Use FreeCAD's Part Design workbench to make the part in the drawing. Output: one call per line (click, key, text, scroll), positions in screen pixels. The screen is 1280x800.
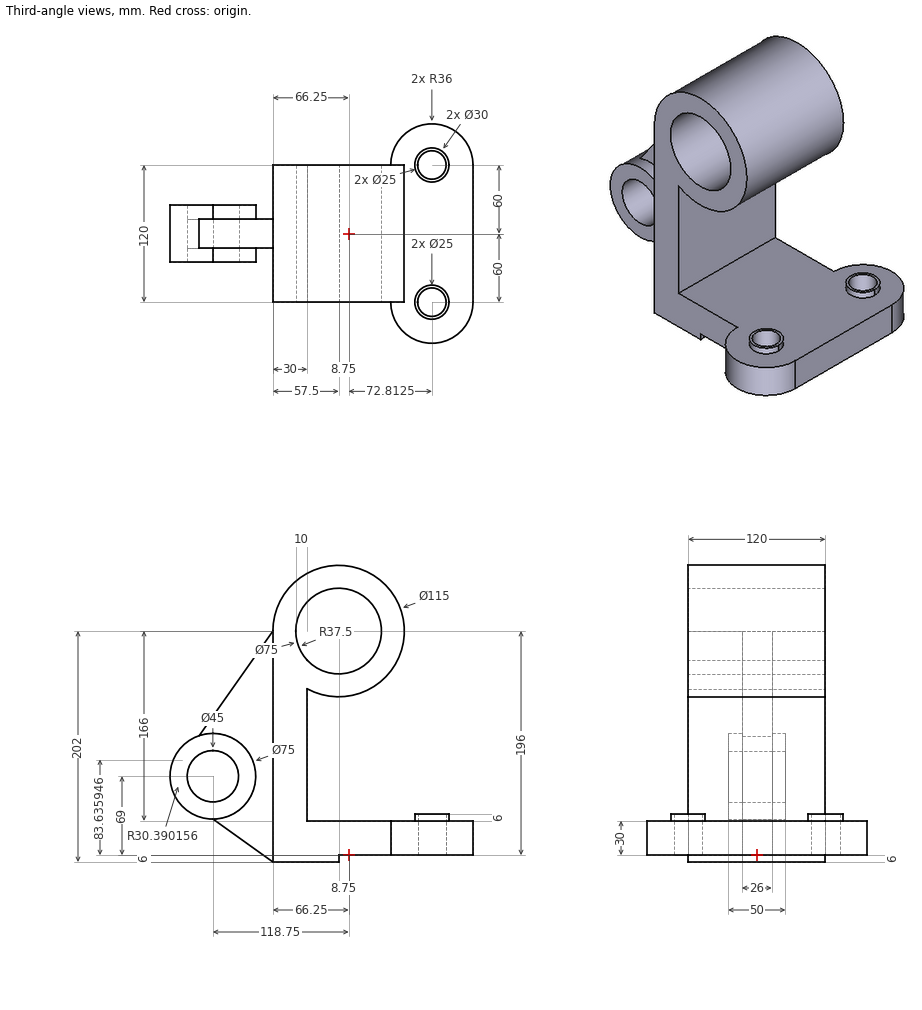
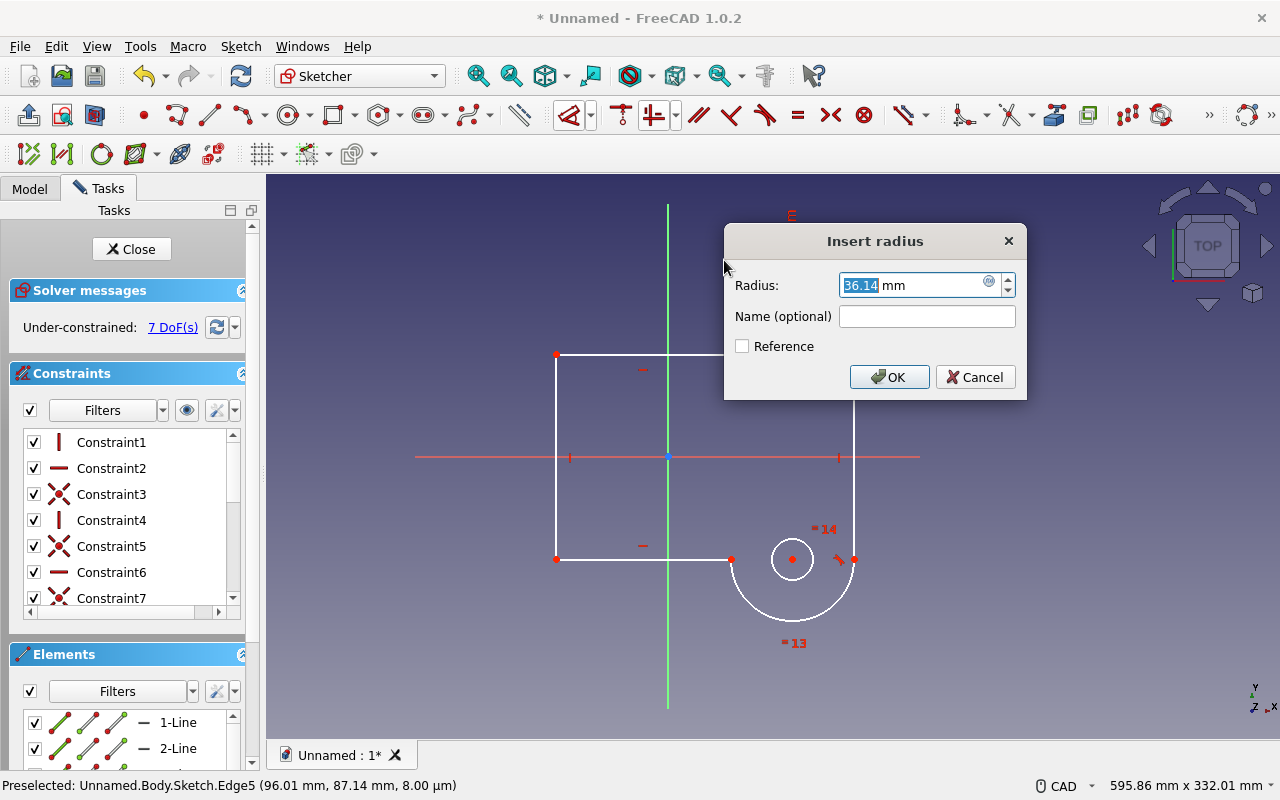
text(36)
key(Return)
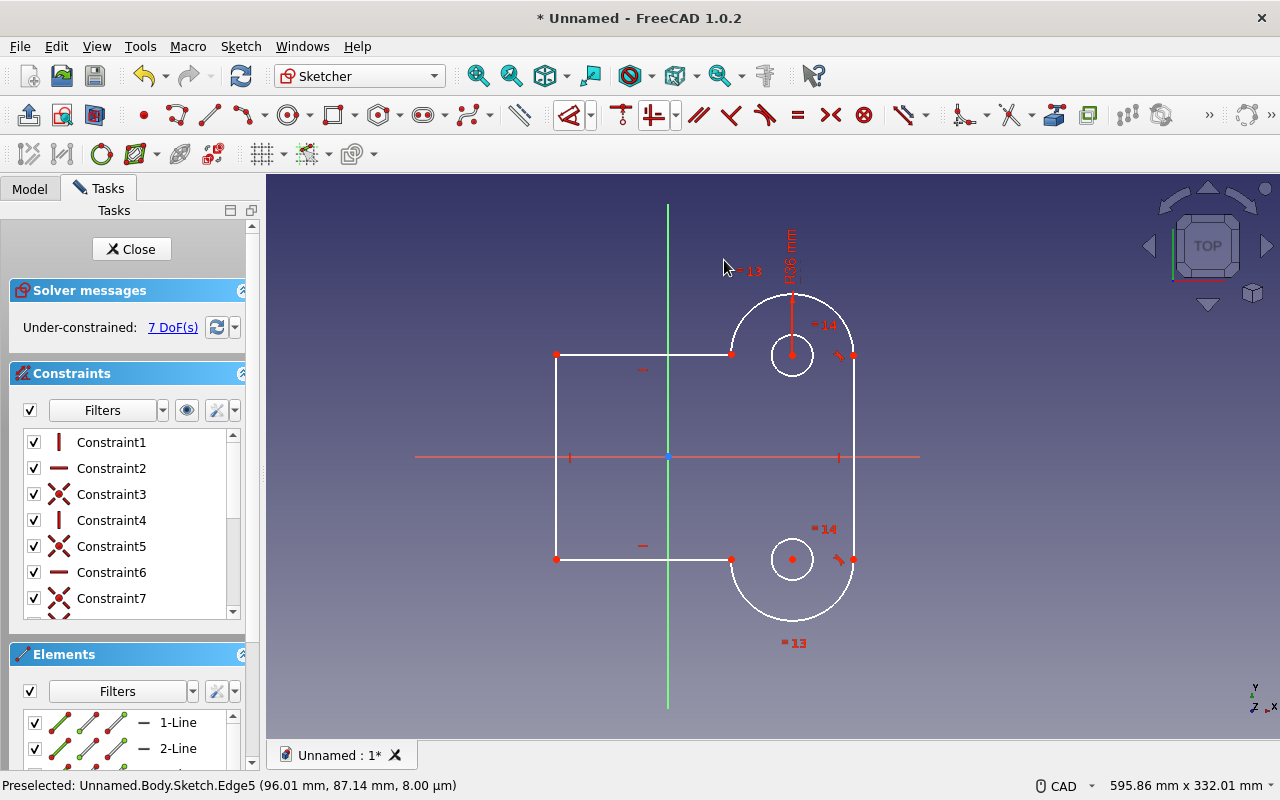
click(807, 545)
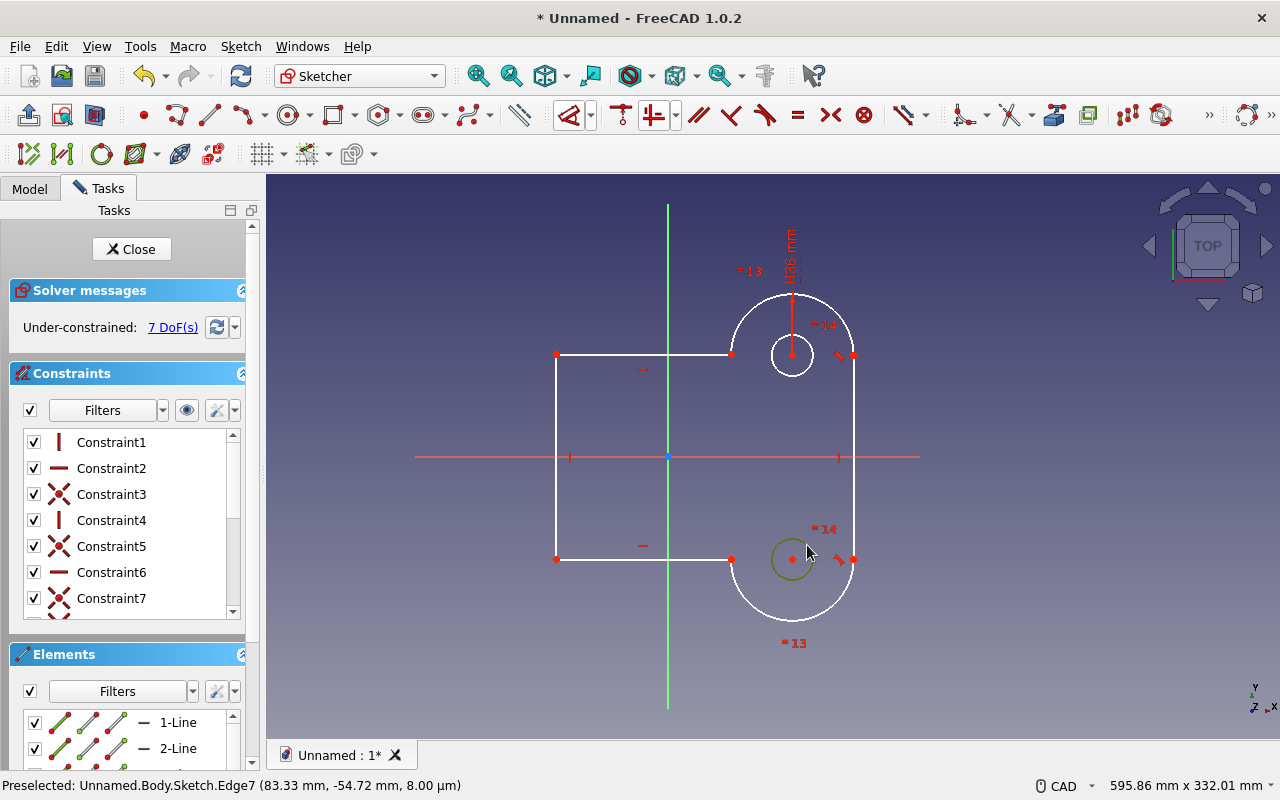
key(k)
key(o)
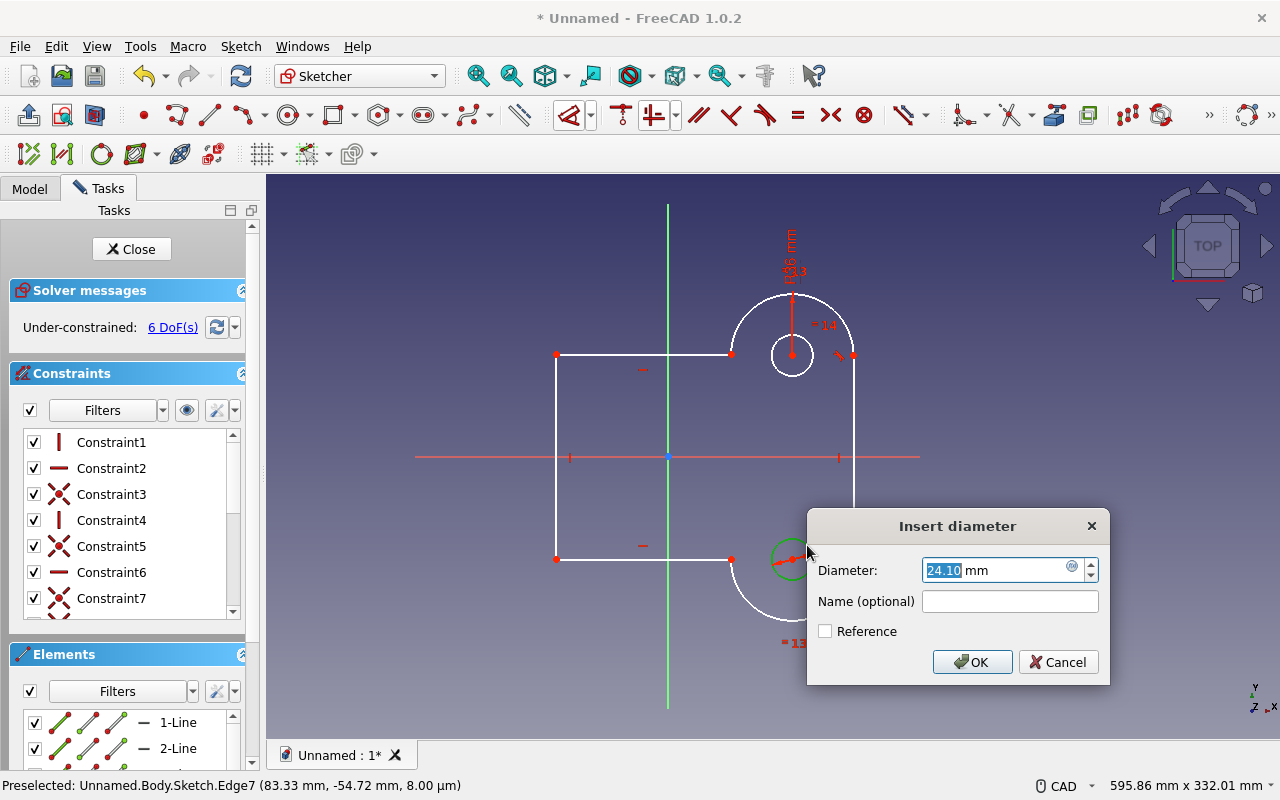
text(25)
key(Return)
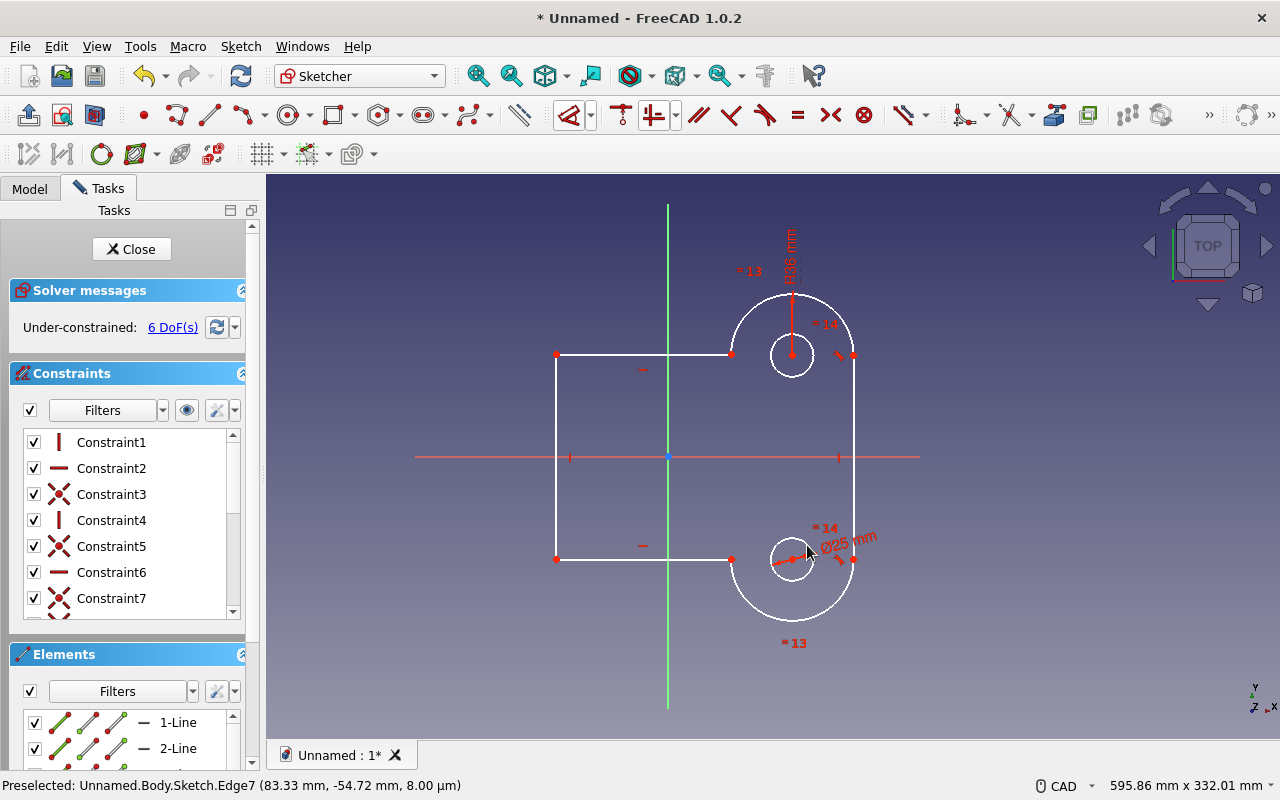
click(792, 560)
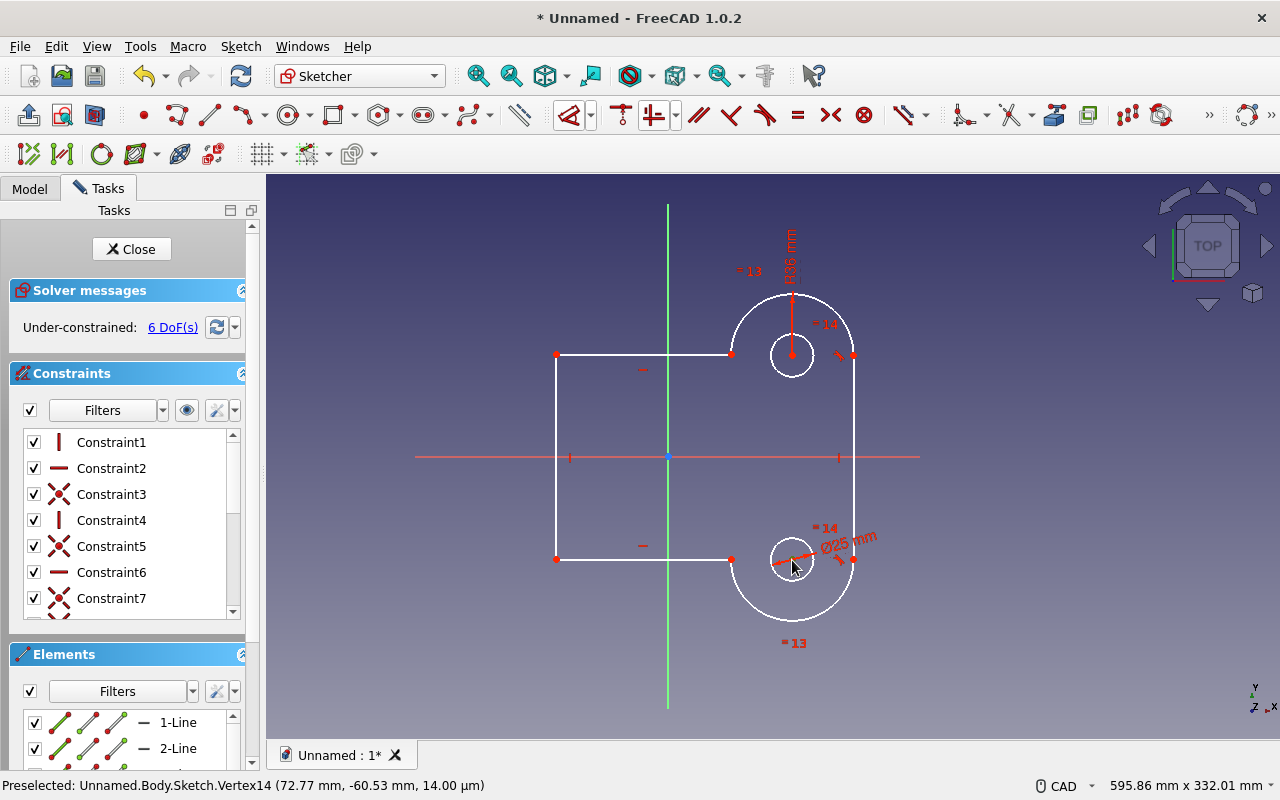
key(i)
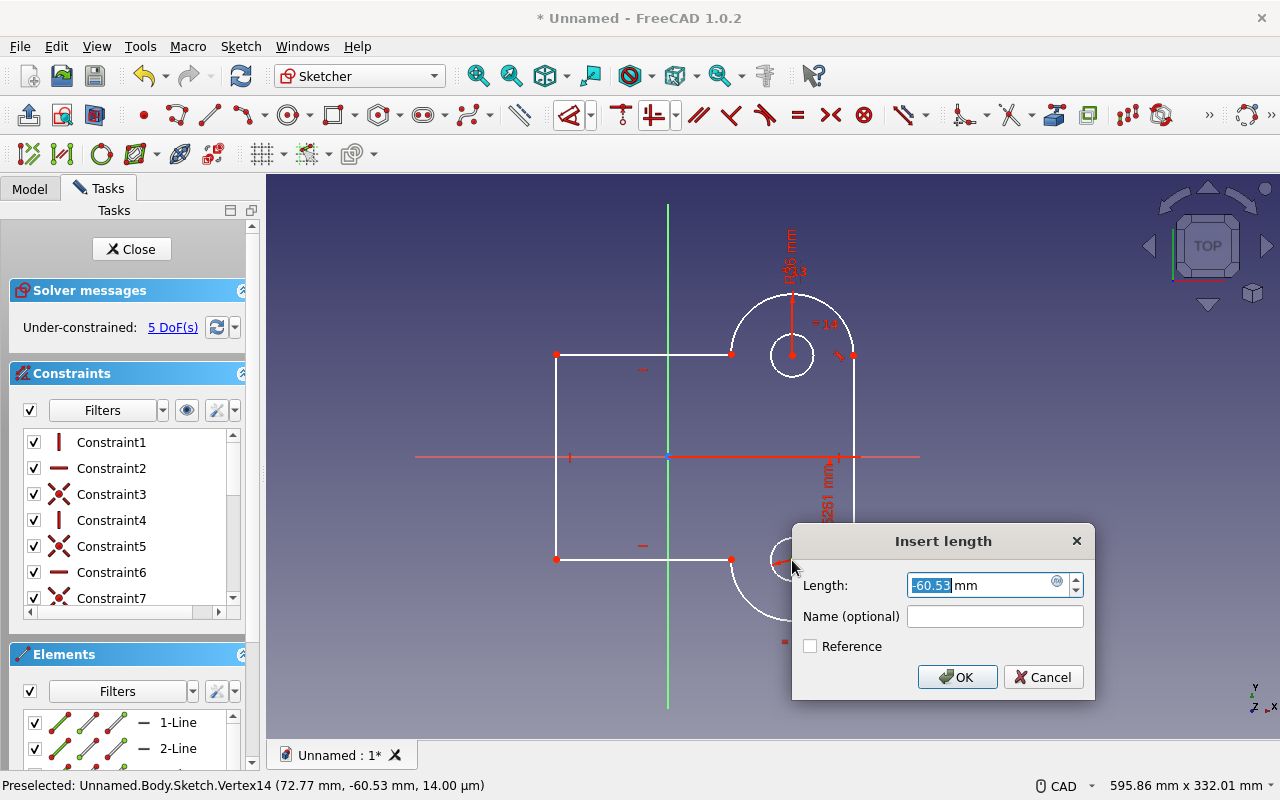
text(-60)
key(Return)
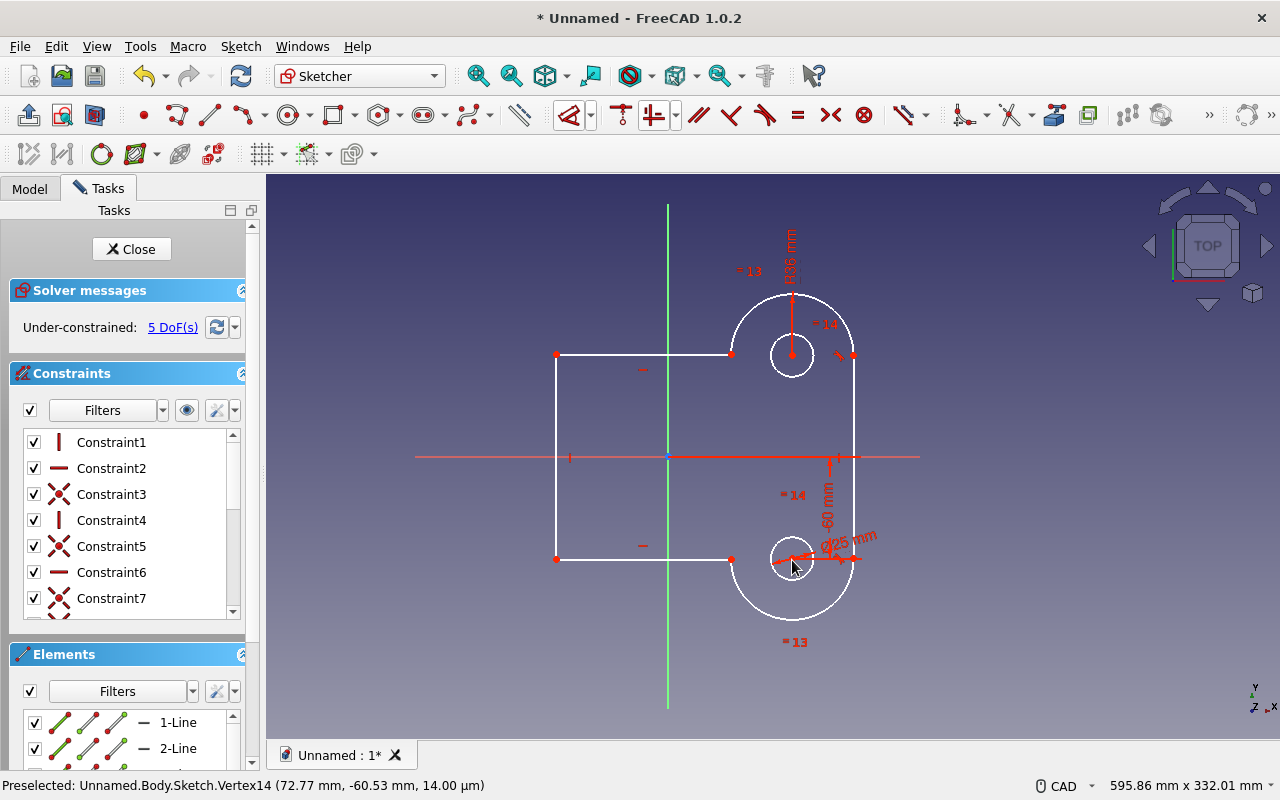
click(792, 356)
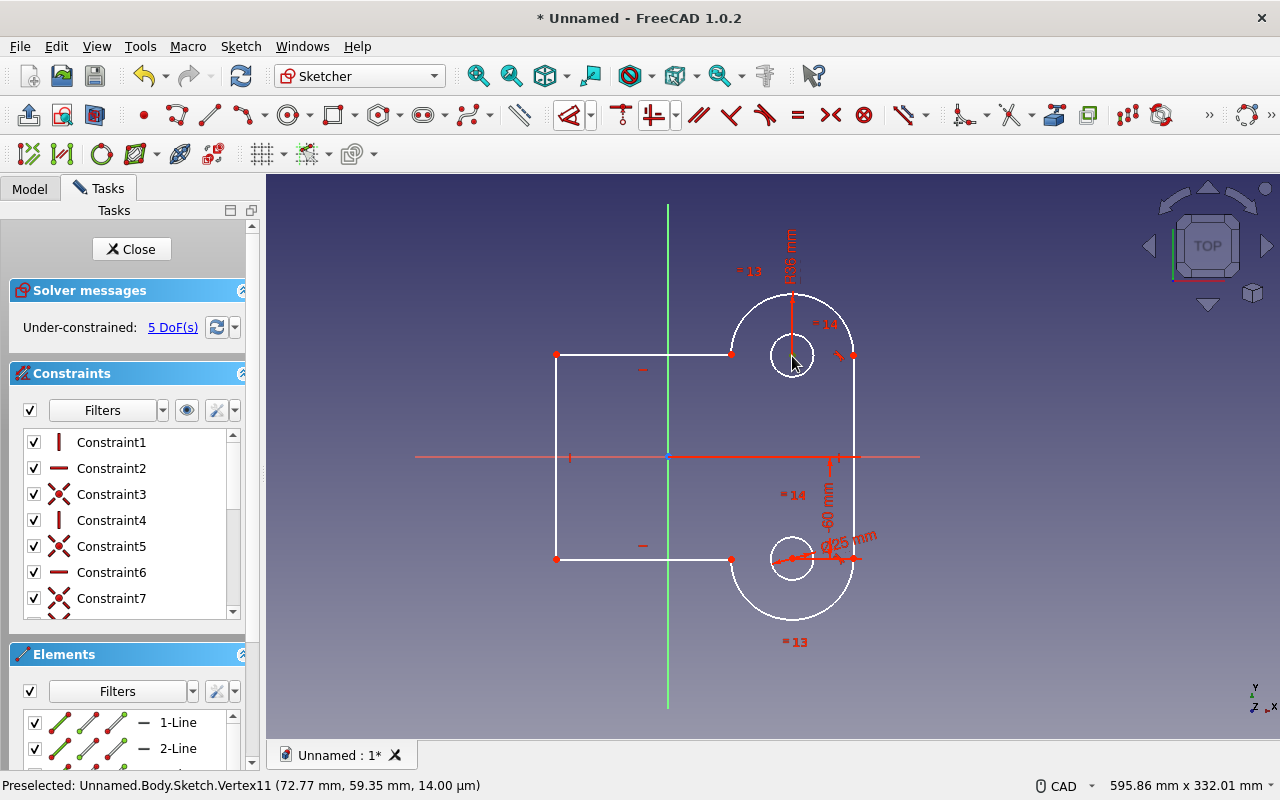
key(i)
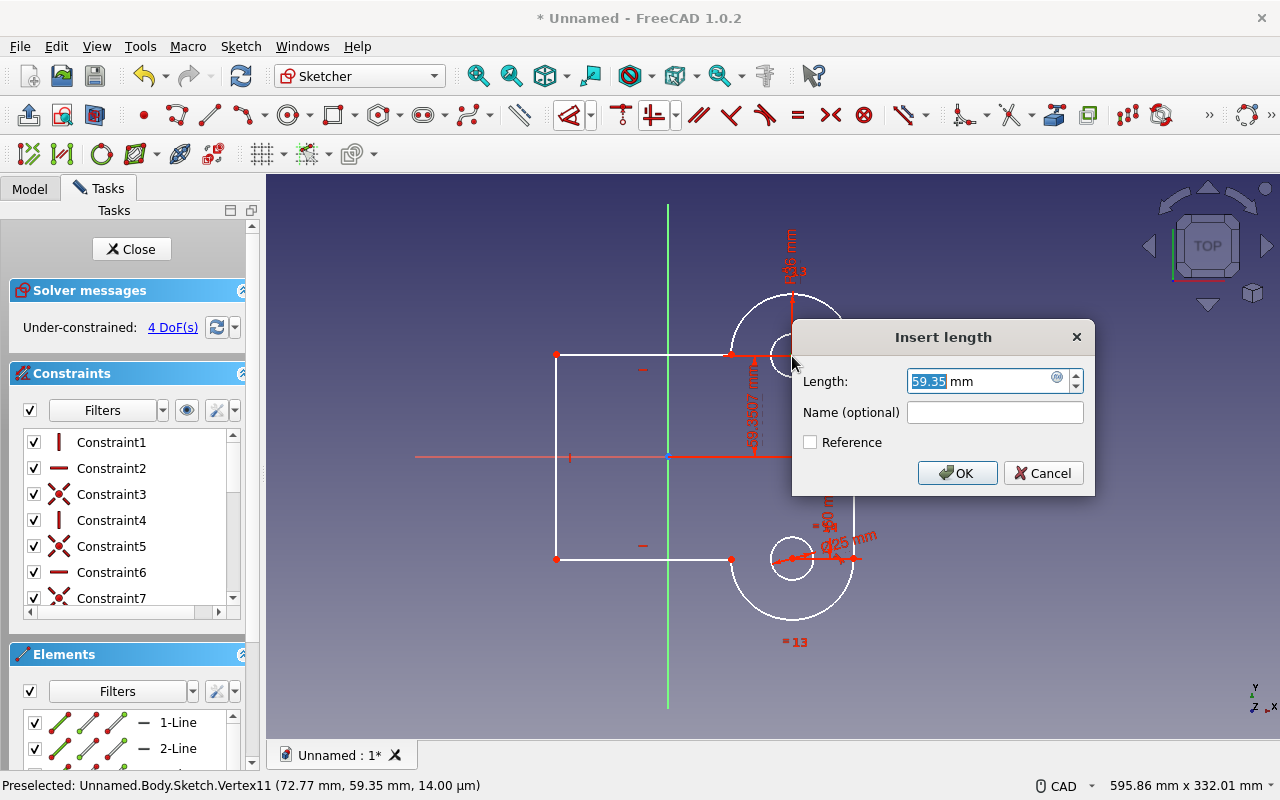
text(60)
key(Return)